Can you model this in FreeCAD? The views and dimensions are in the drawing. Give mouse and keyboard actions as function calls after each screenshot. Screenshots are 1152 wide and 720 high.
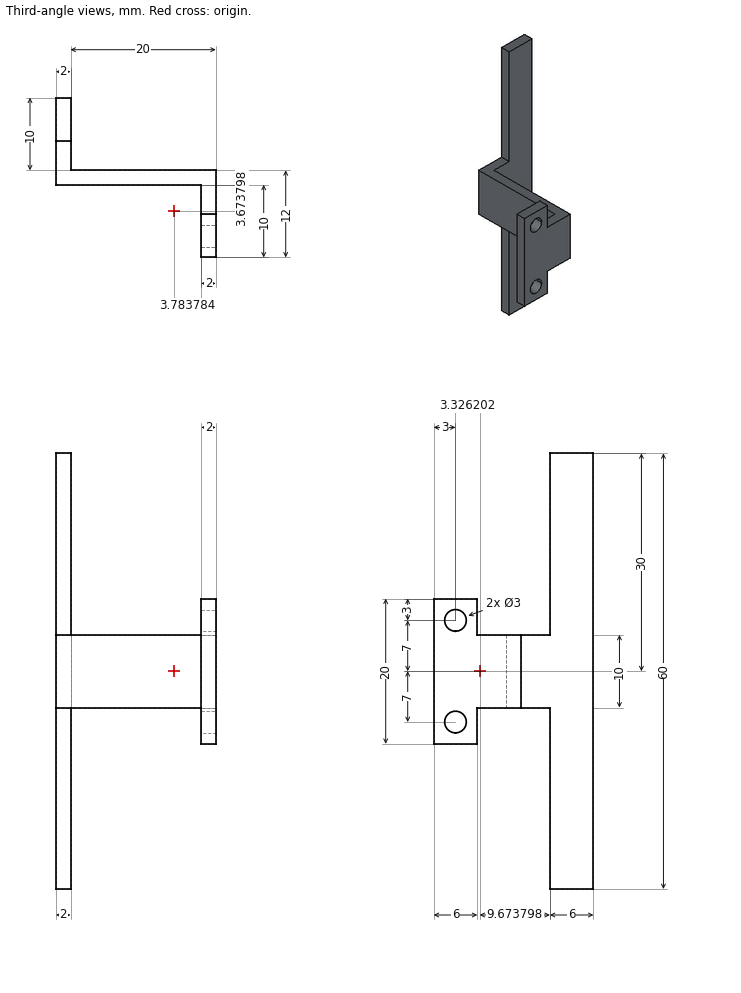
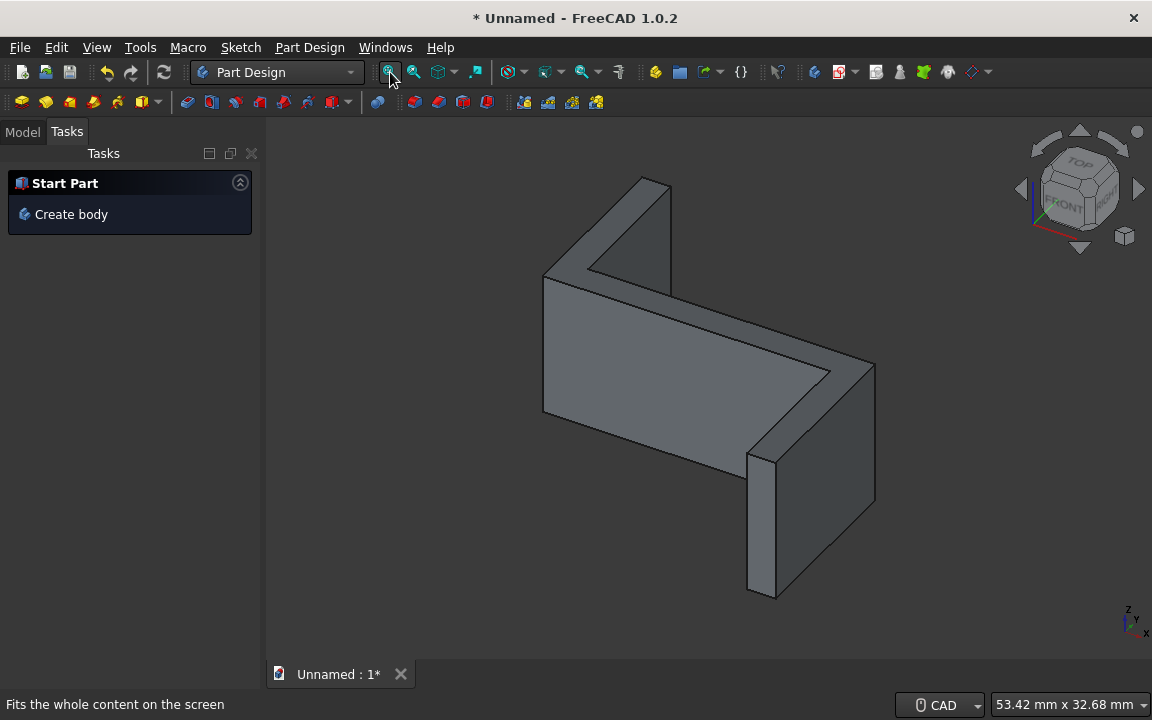
click(826, 481)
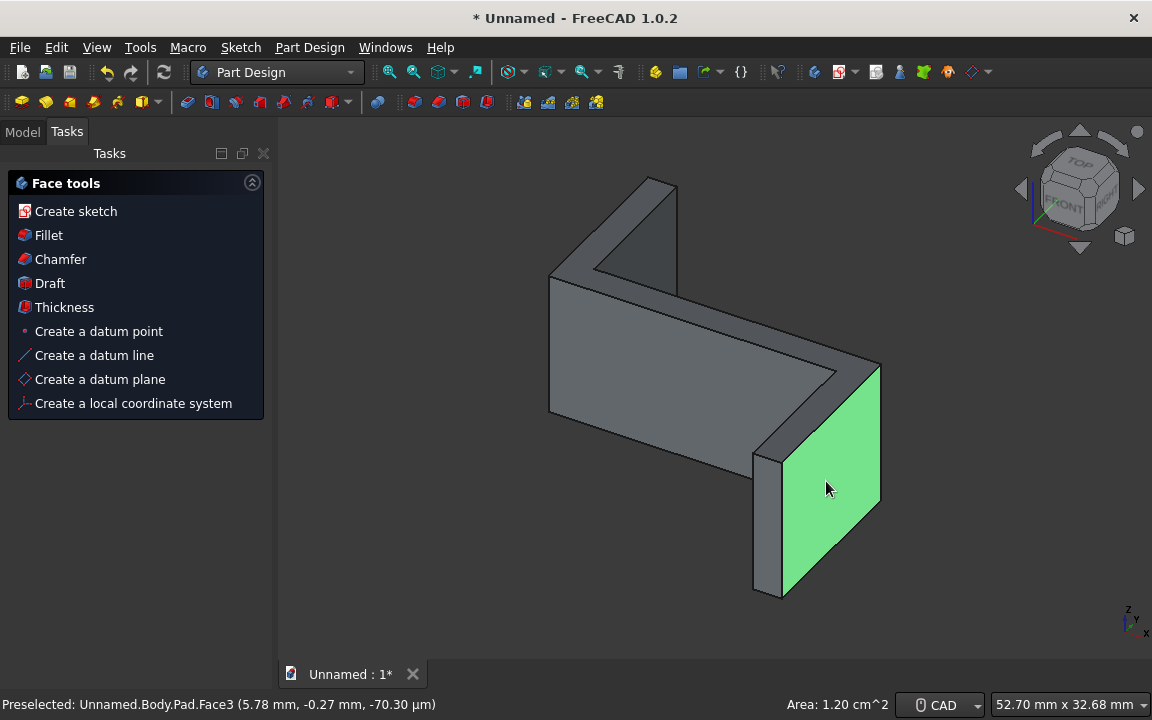
click(840, 72)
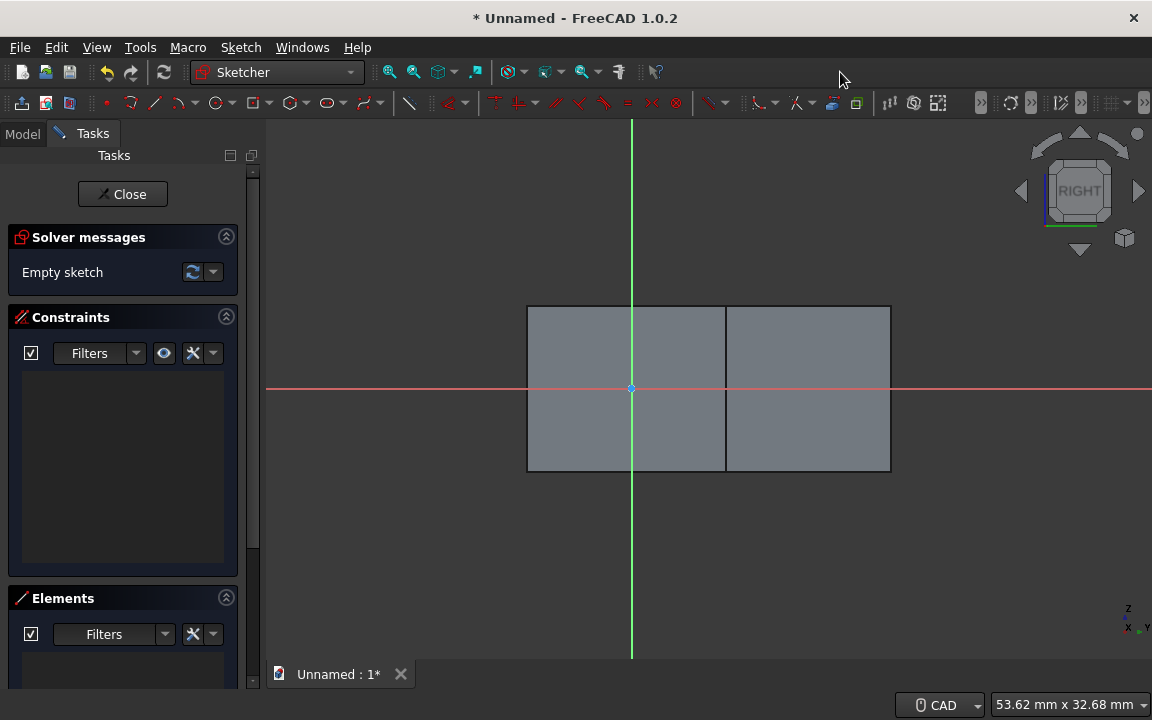
key(g)
key(r)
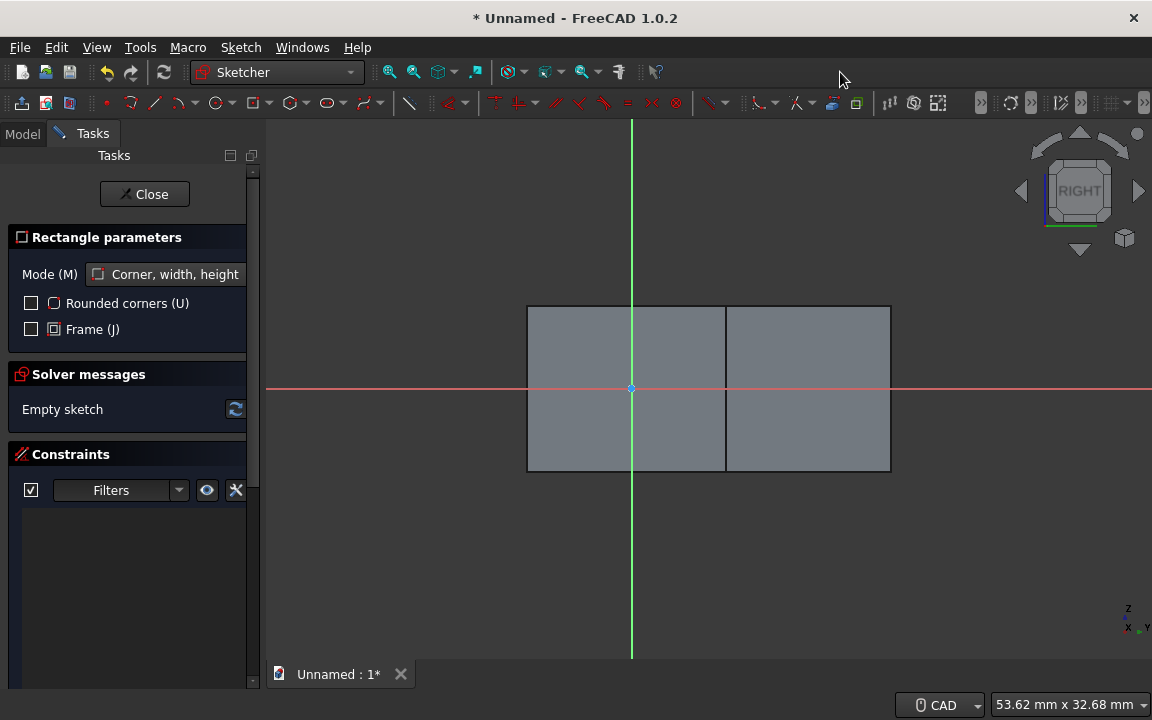
click(527, 224)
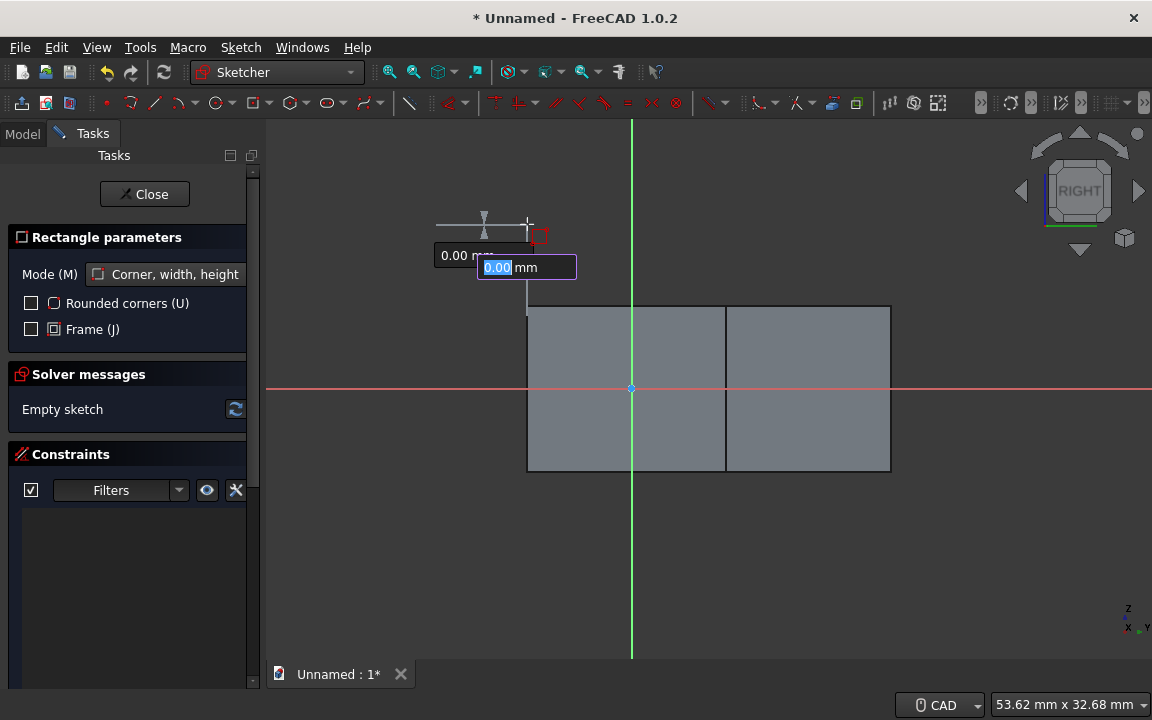
scroll(626, 554, up, 6)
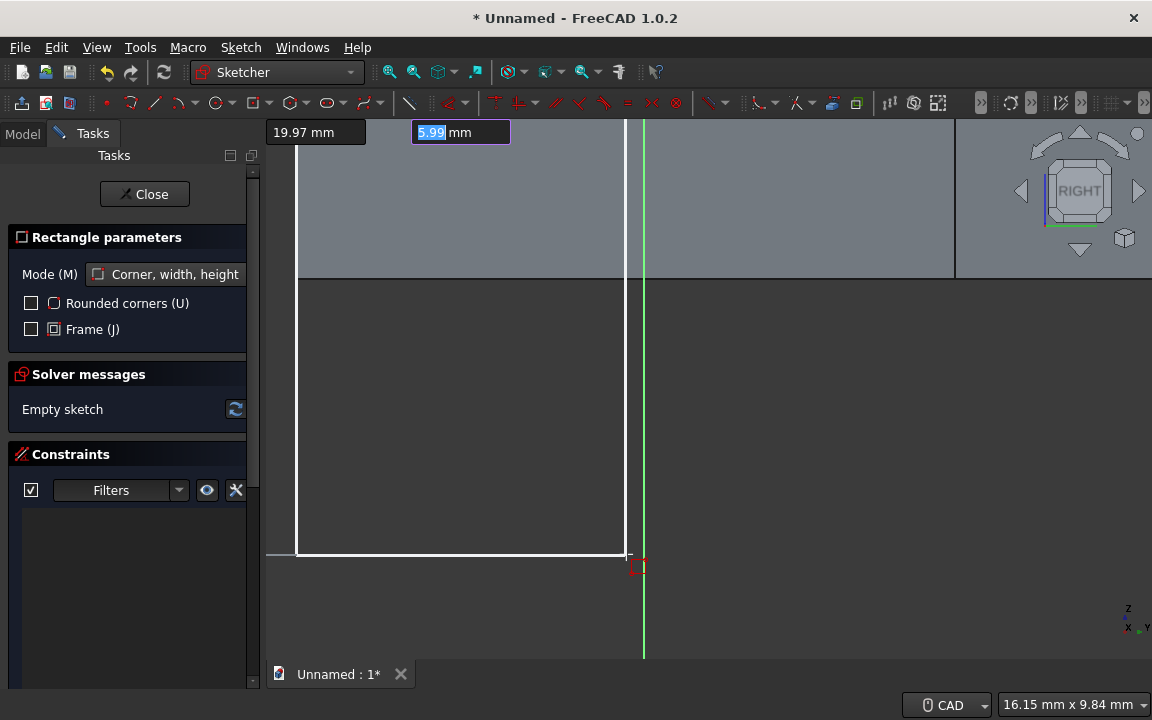
click(626, 553)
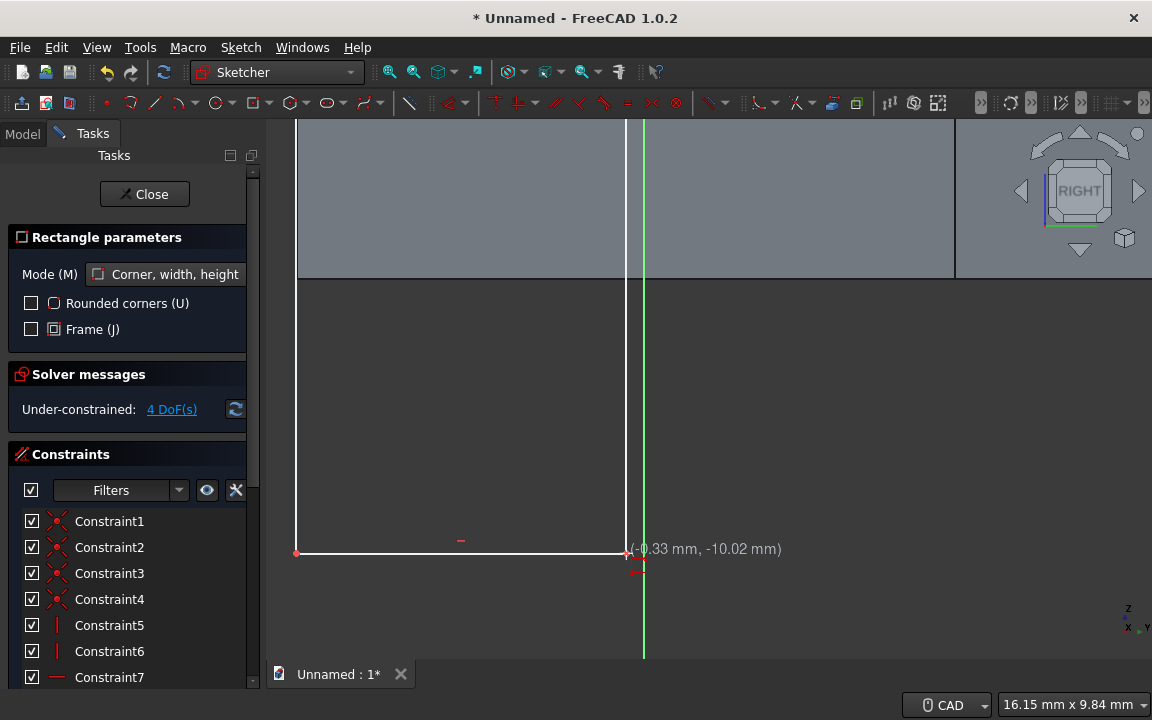
click(216, 104)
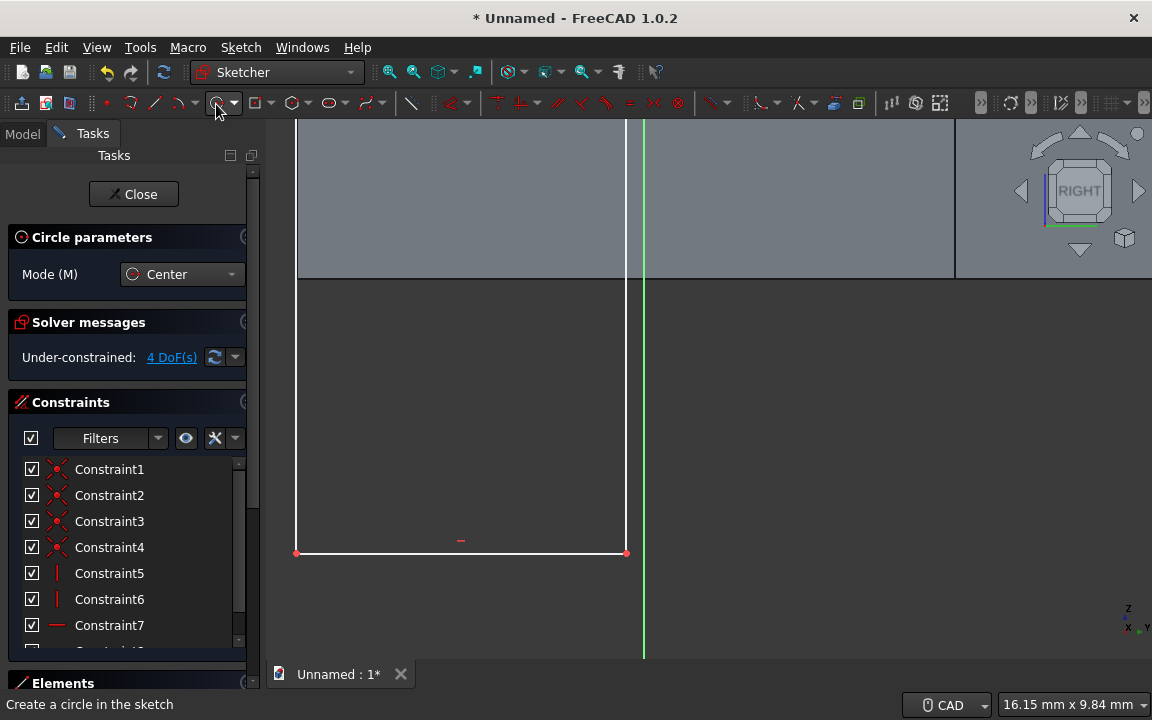
scroll(714, 555, down, 6)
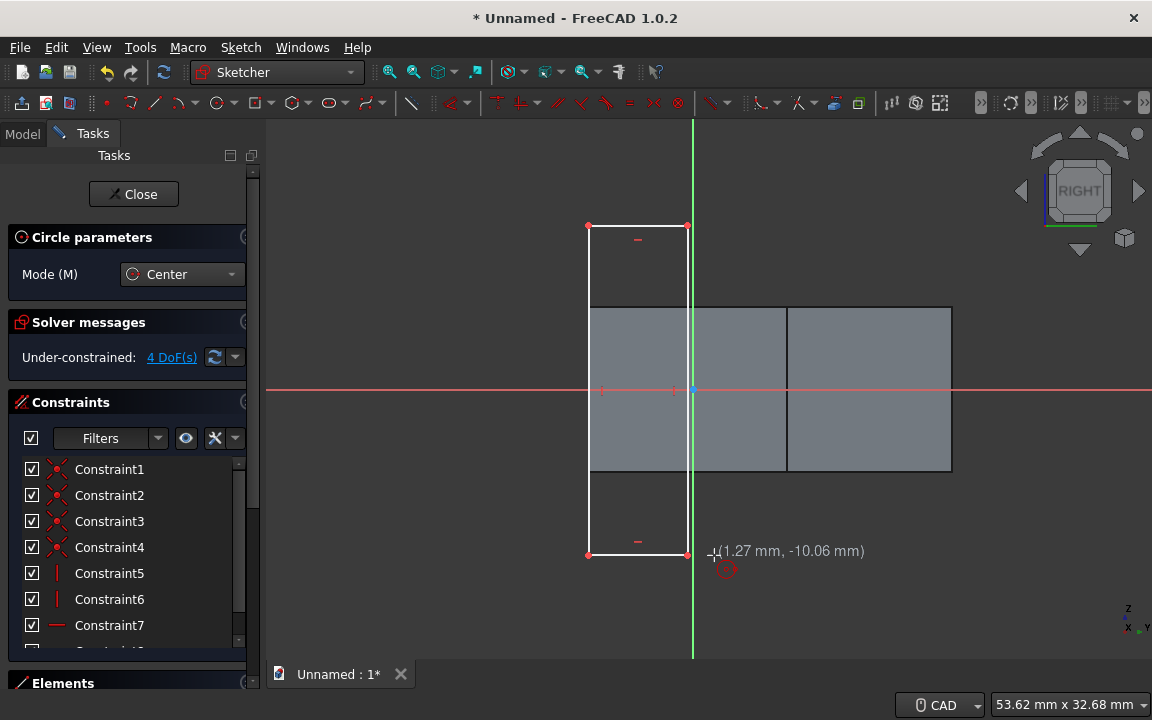
click(638, 274)
click(656, 257)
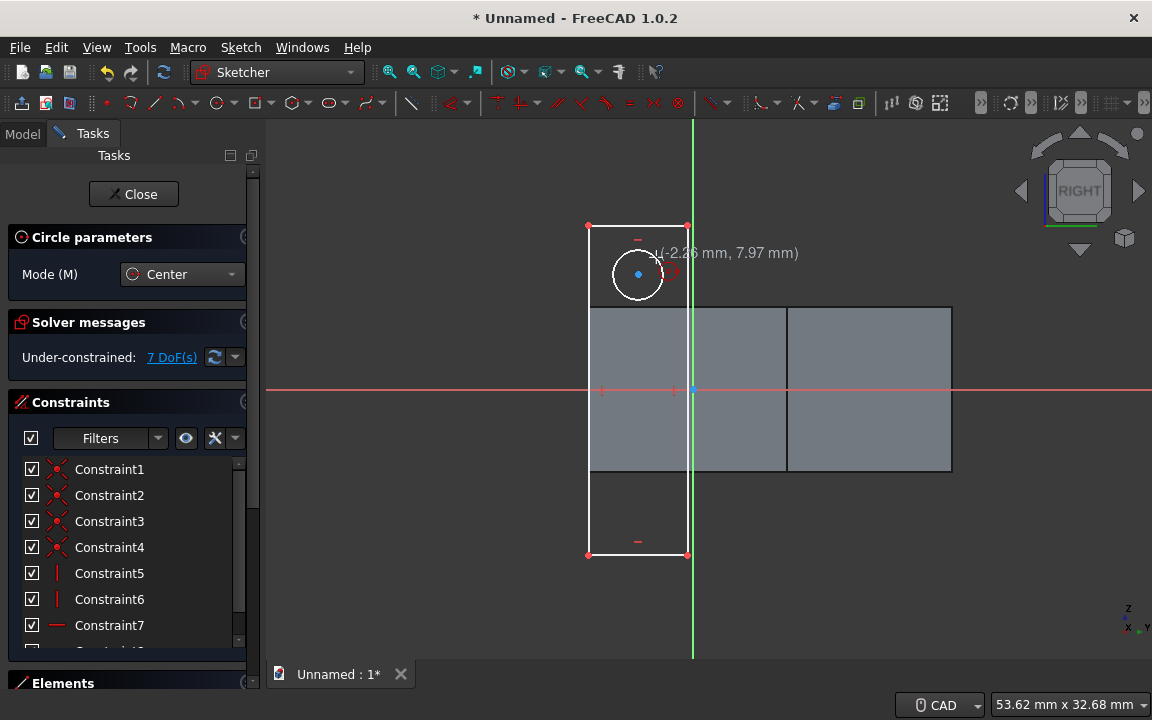
click(638, 505)
click(656, 488)
key(Escape)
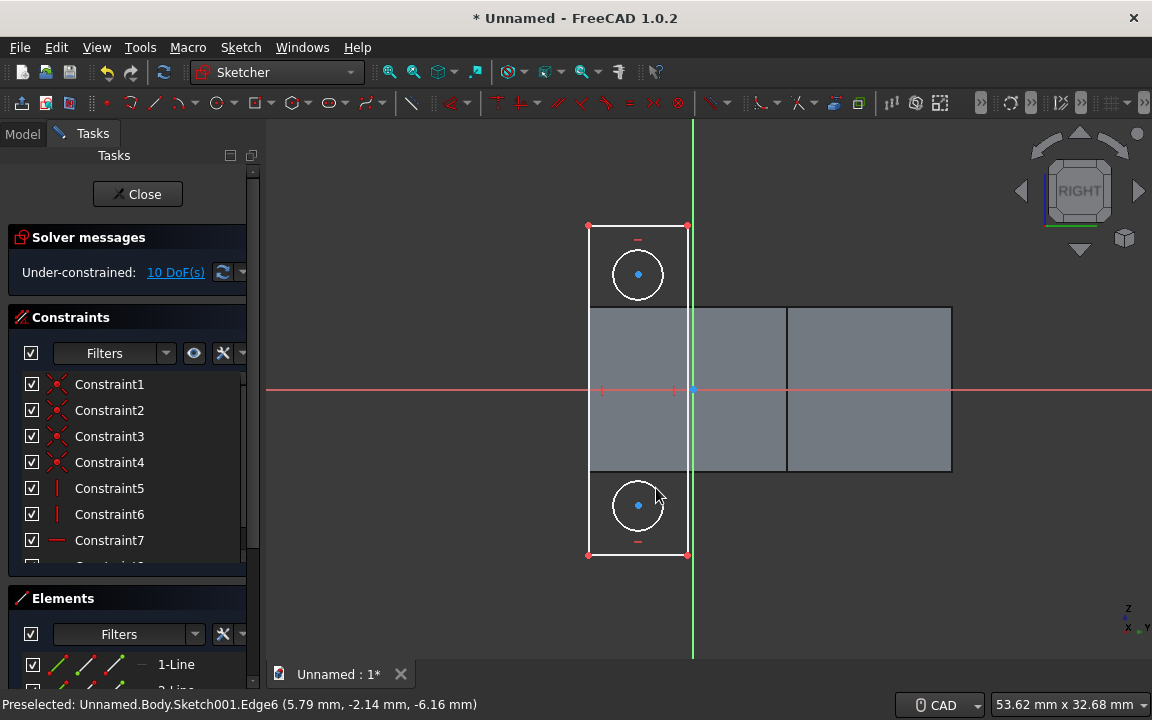
click(655, 257)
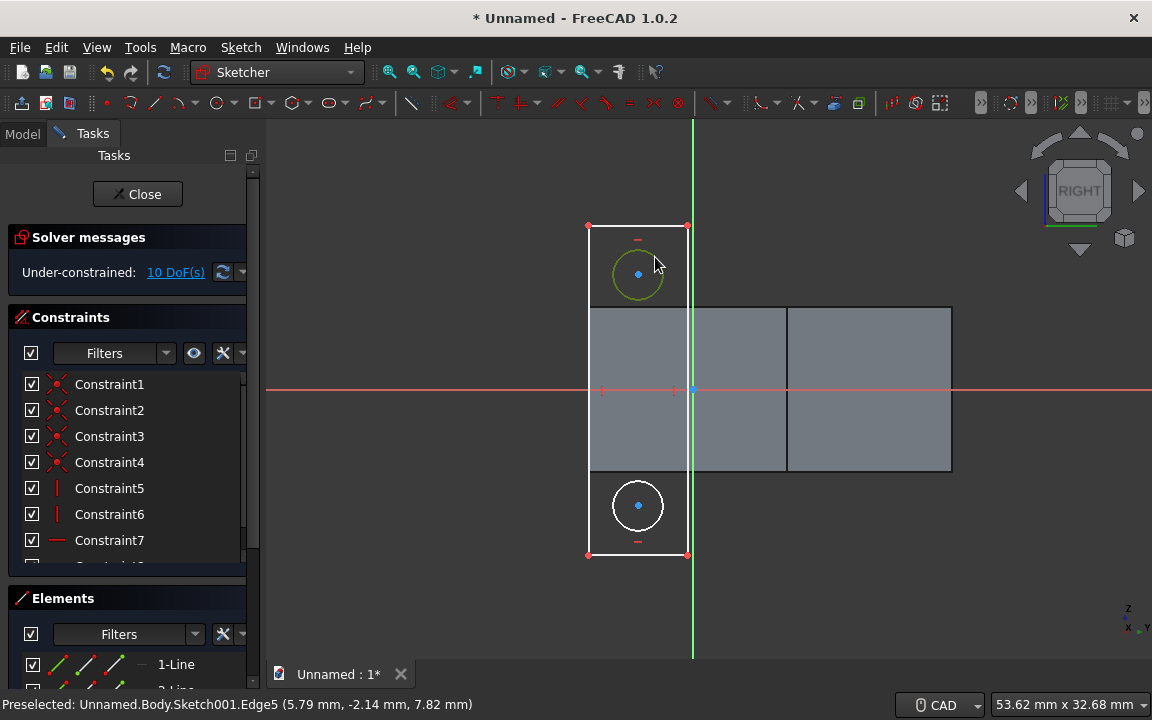
click(655, 488)